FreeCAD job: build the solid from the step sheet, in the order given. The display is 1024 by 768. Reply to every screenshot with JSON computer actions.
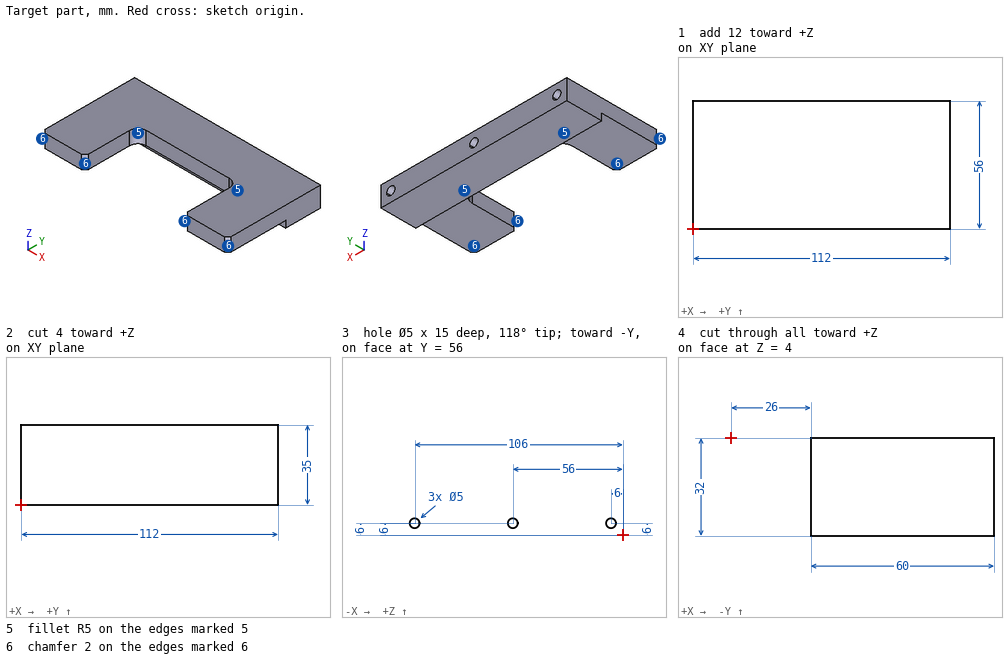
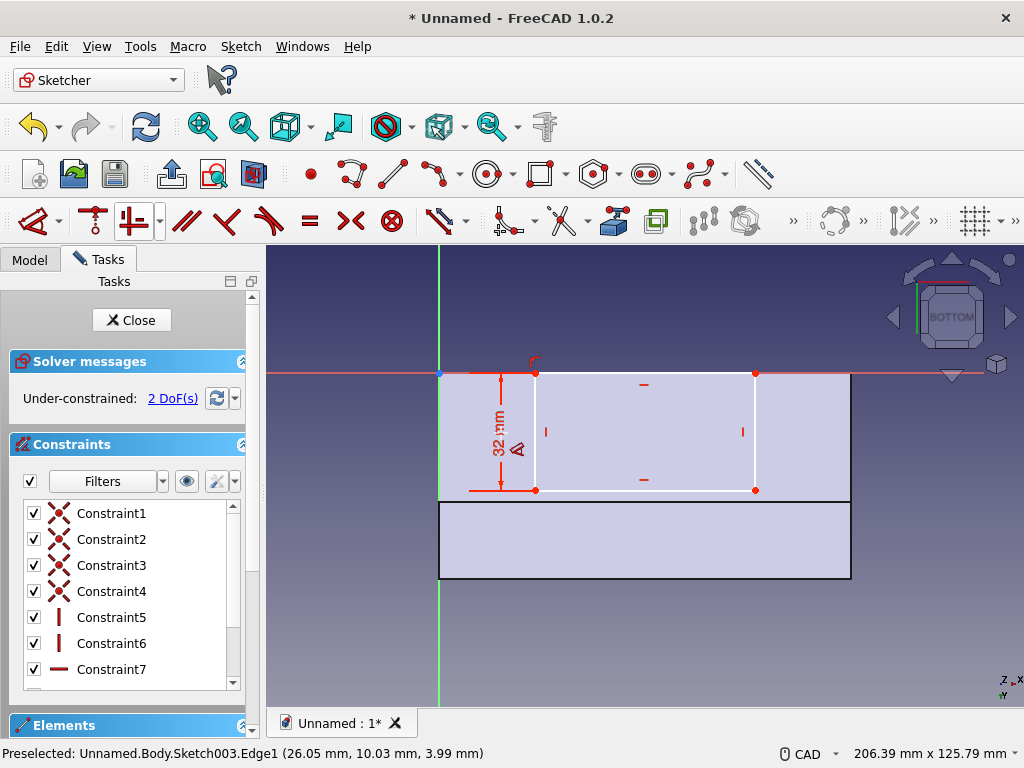
{"action": "left_click", "coordinate": [601, 491]}
{"action": "left_click", "coordinate": [645, 525]}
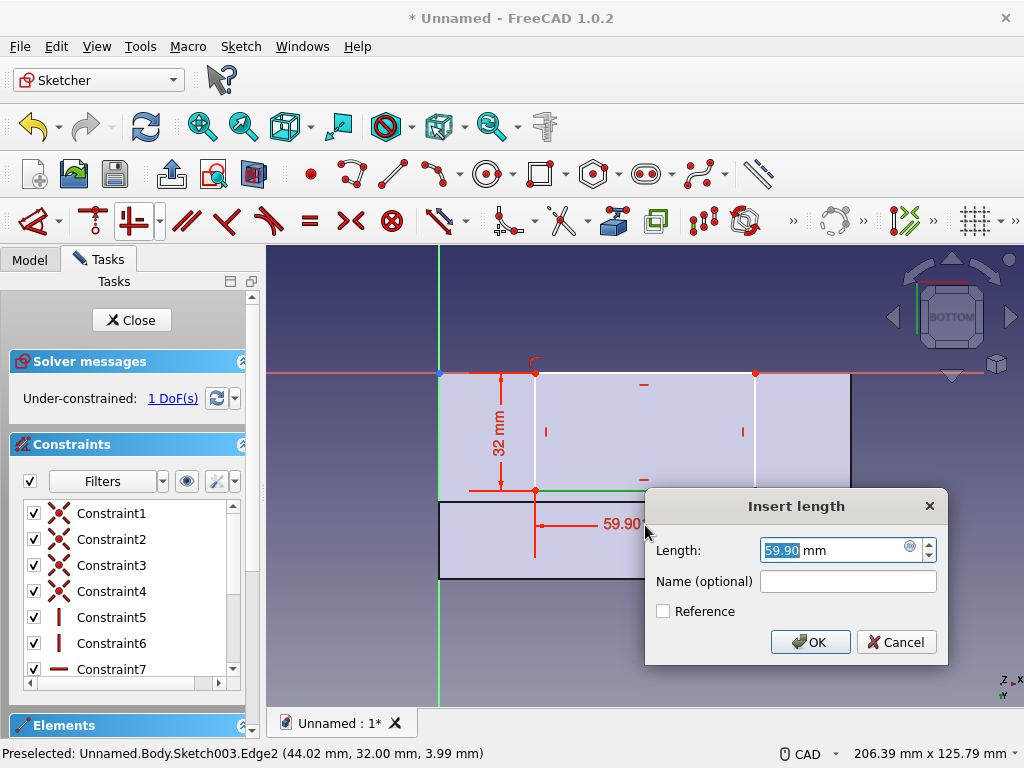
{"action": "type", "text": "60"}
{"action": "key", "text": "Return"}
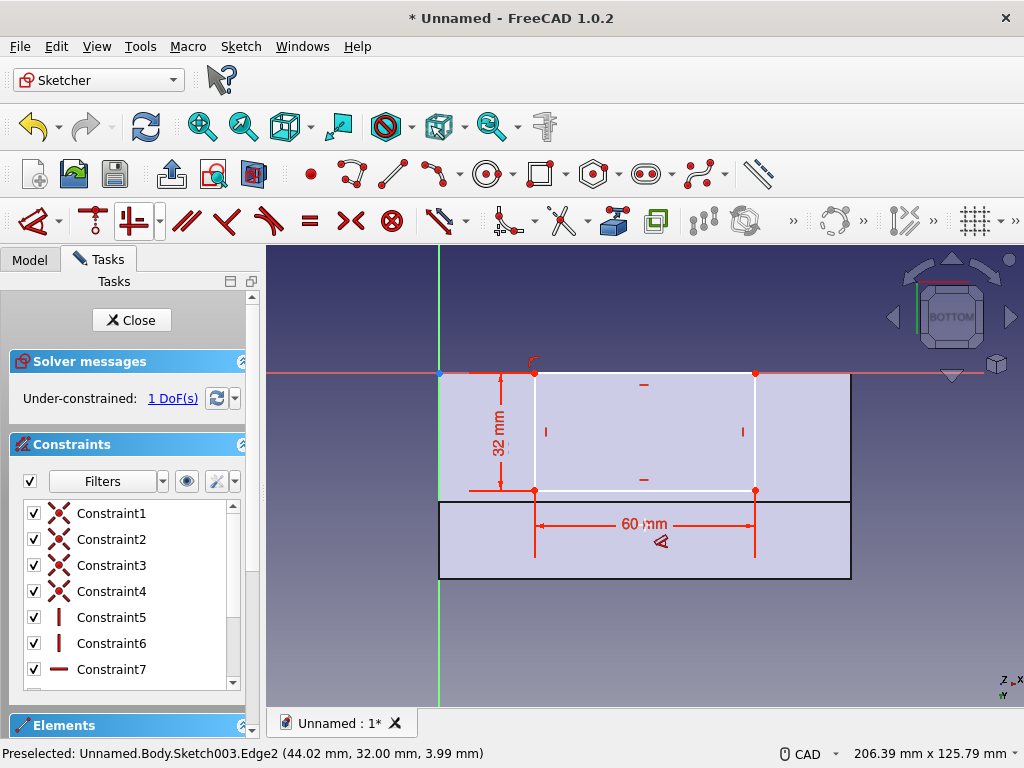
{"action": "left_click", "coordinate": [535, 373]}
{"action": "left_click", "coordinate": [487, 339]}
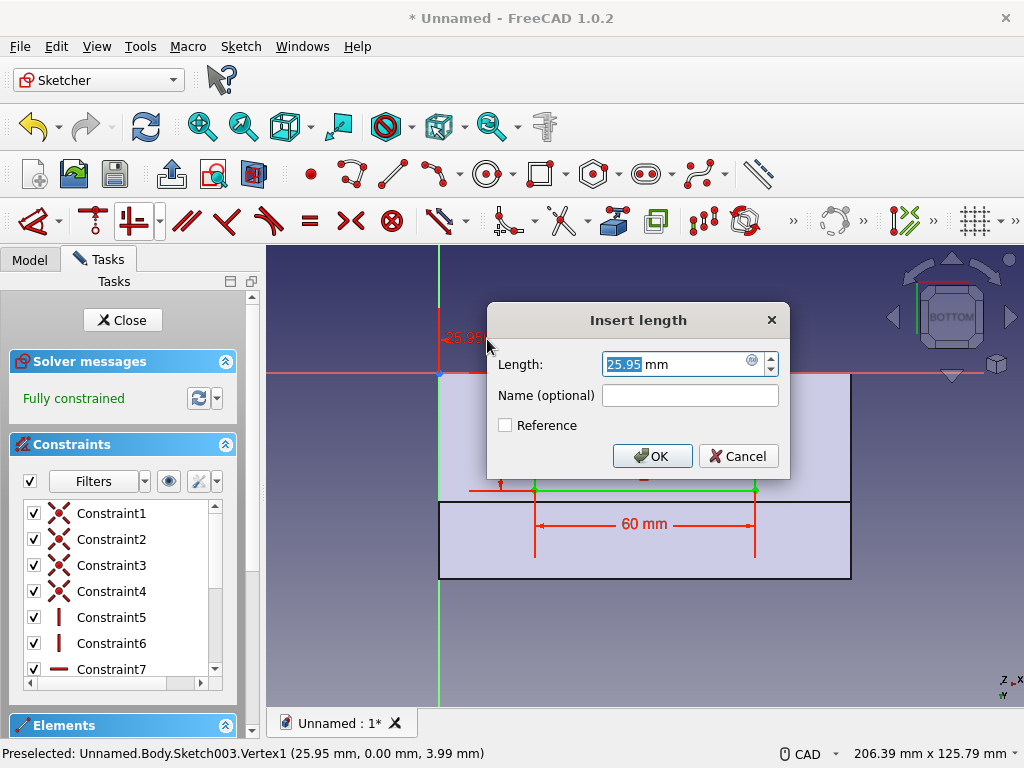
{"action": "type", "text": "26"}
{"action": "key", "text": "Return"}
{"action": "key", "text": "Escape"}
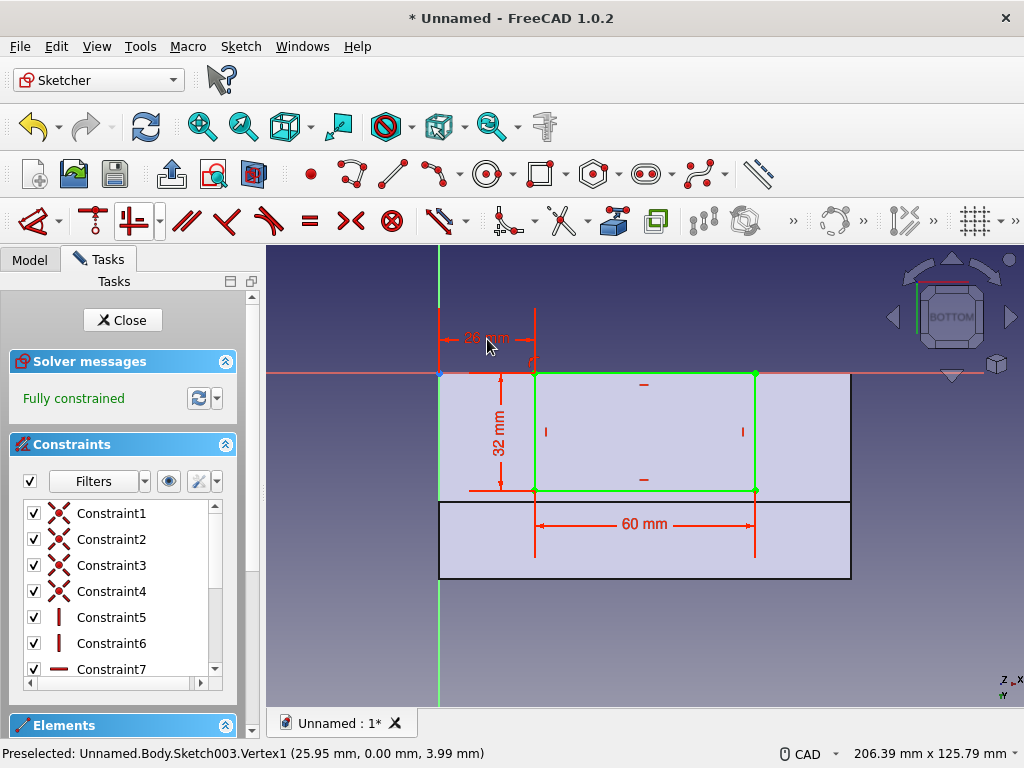
{"action": "left_click", "coordinate": [123, 320]}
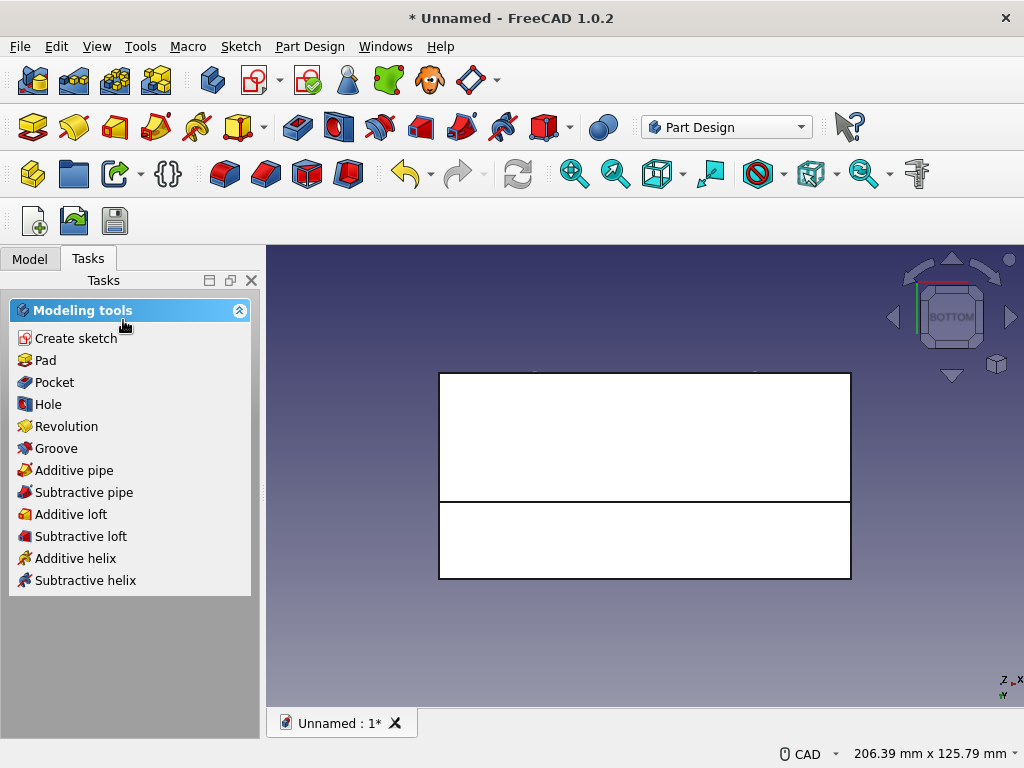
{"action": "left_click", "coordinate": [298, 128]}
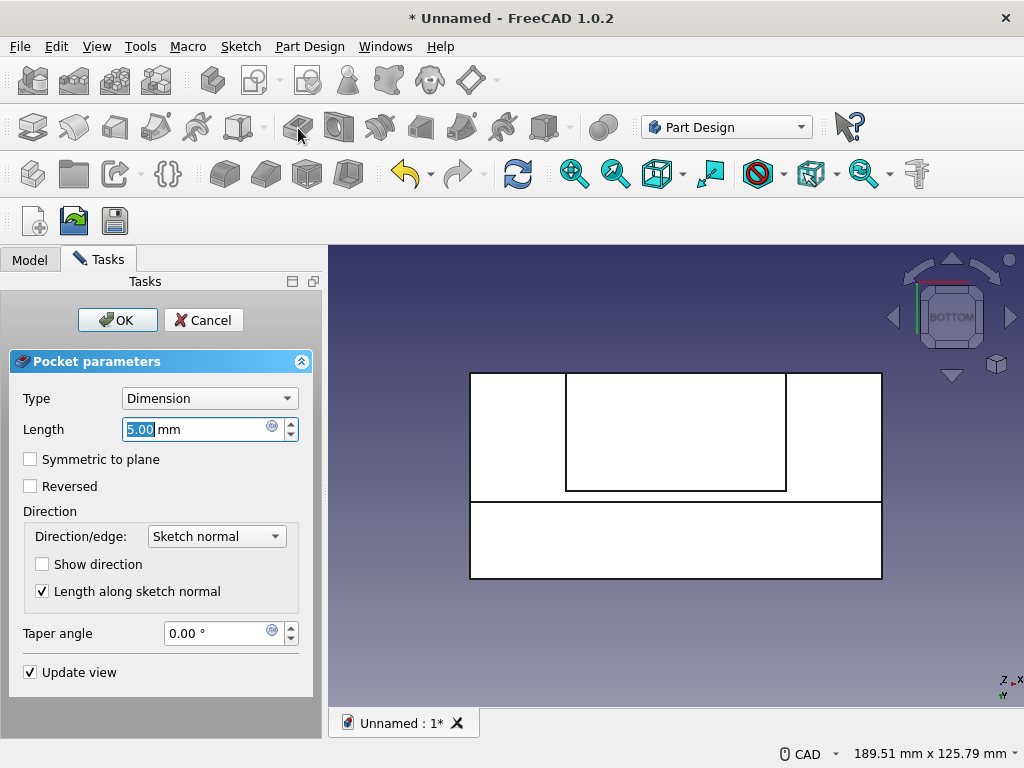
{"action": "left_click", "coordinate": [210, 398]}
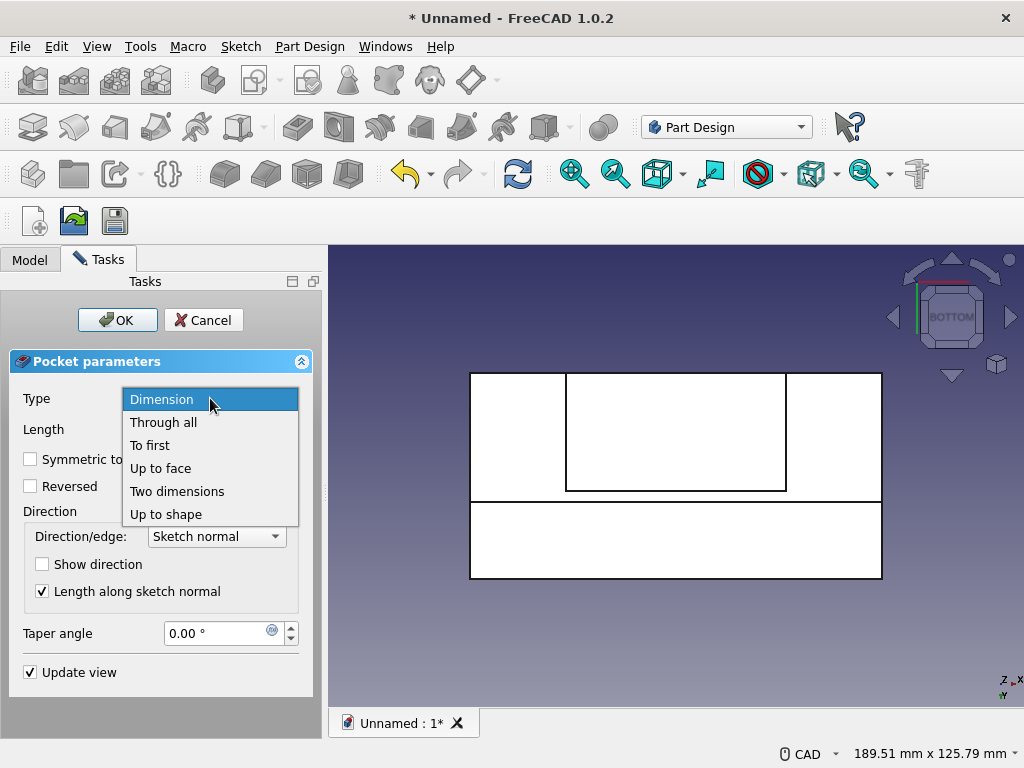
{"action": "left_click", "coordinate": [208, 422]}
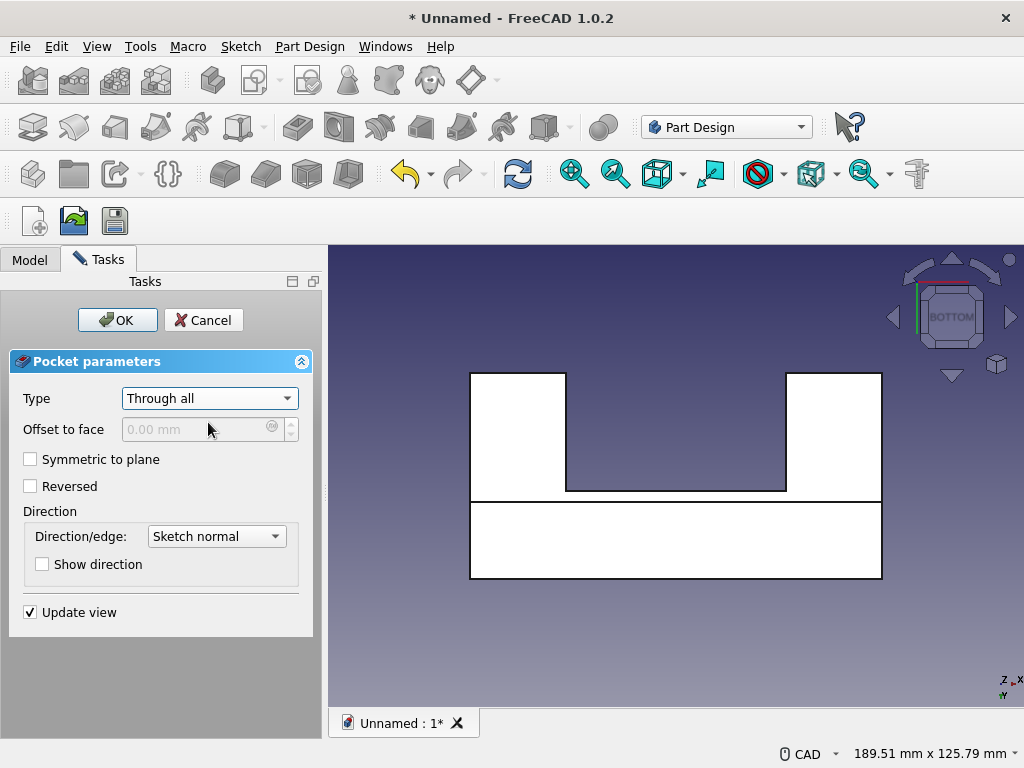
{"action": "left_click", "coordinate": [118, 320]}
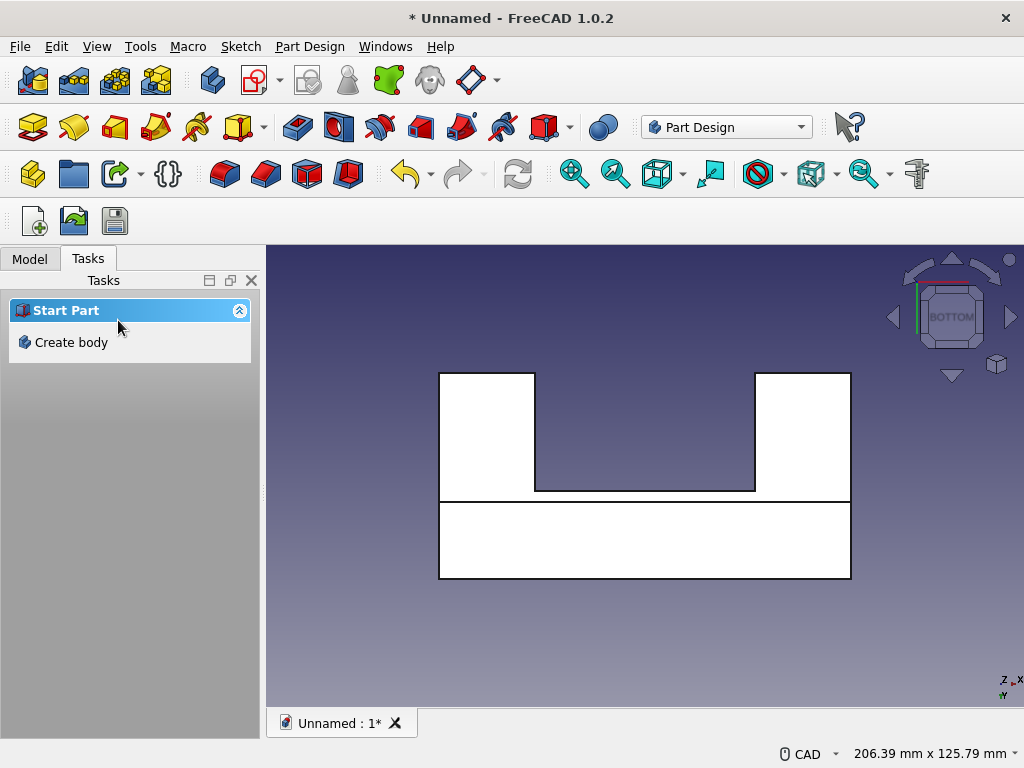
{"action": "key", "text": "0"}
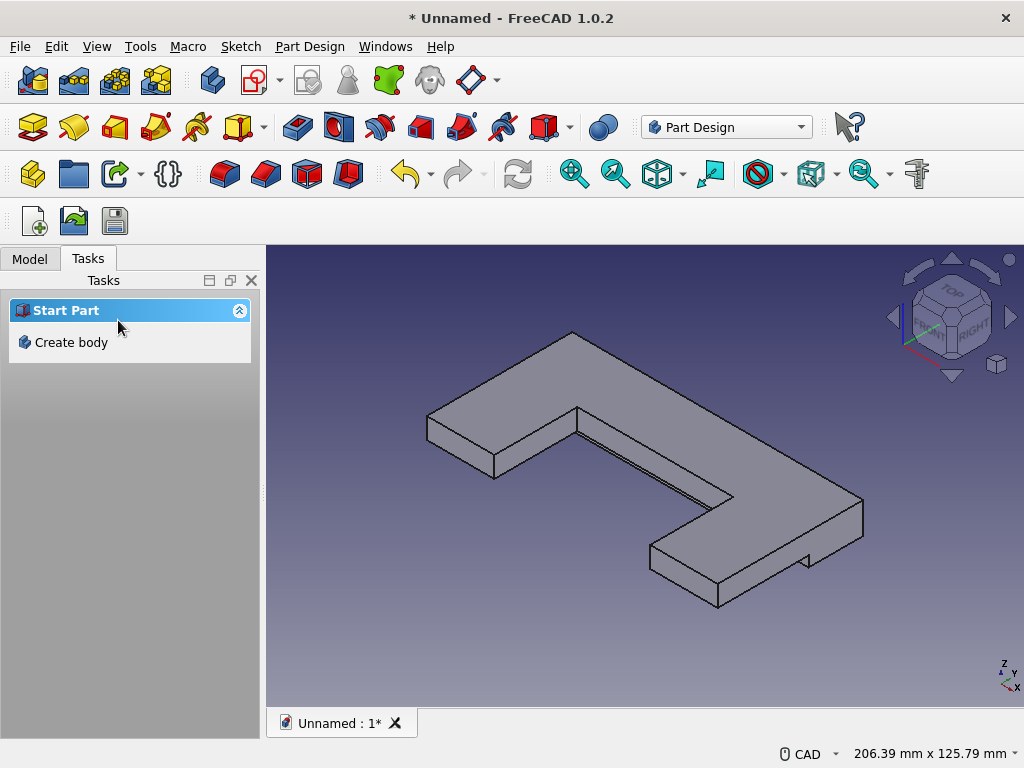
{"action": "key", "text": "2"}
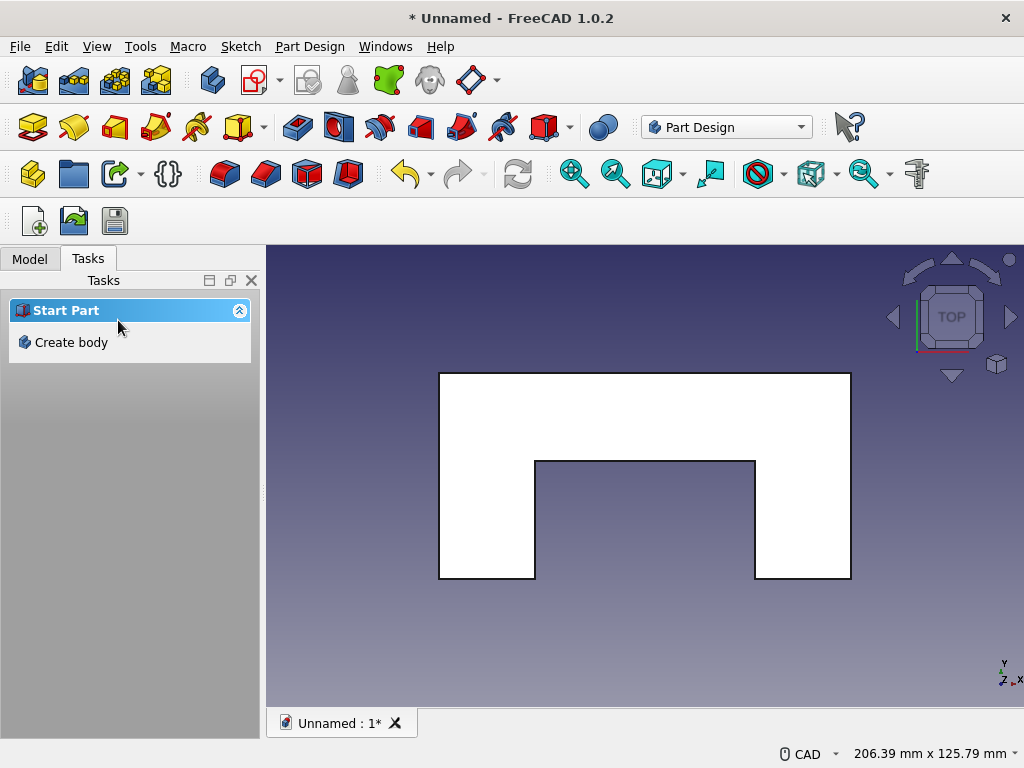
{"action": "key", "text": "1"}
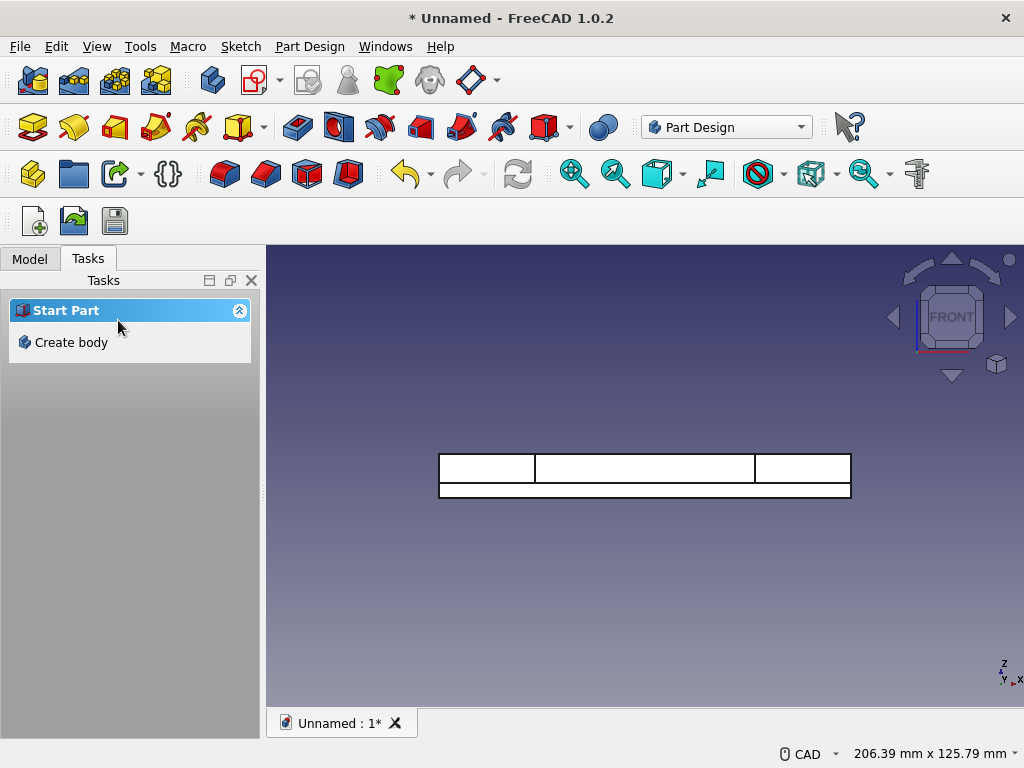
{"action": "key", "text": "3"}